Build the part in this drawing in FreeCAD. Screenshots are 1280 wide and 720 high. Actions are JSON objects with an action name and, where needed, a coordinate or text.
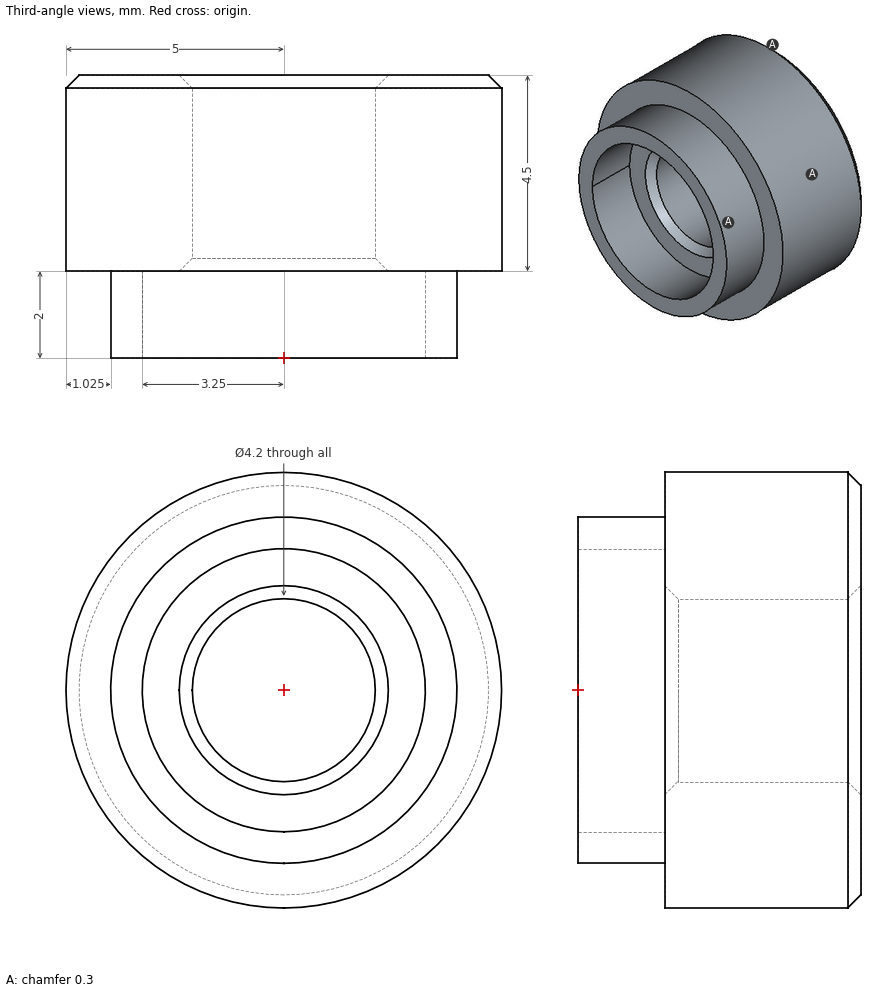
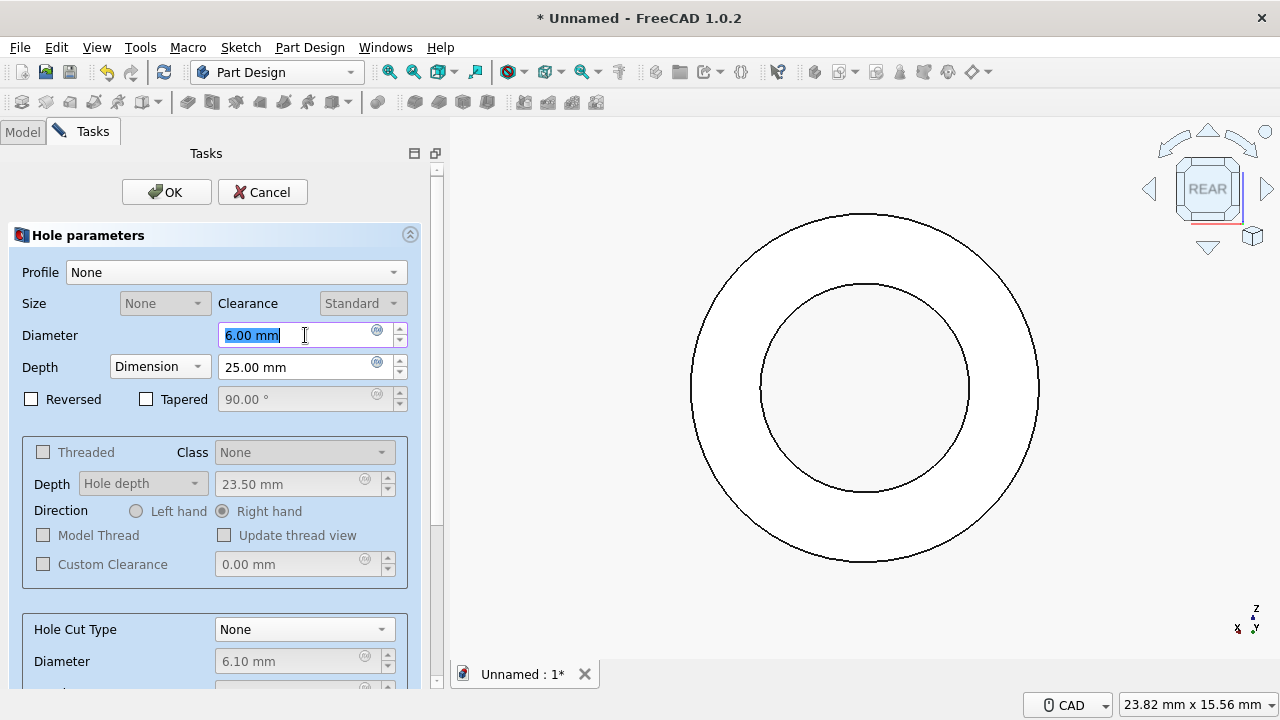
{"action": "type", "text": "4.2"}
{"action": "key", "text": "Tab"}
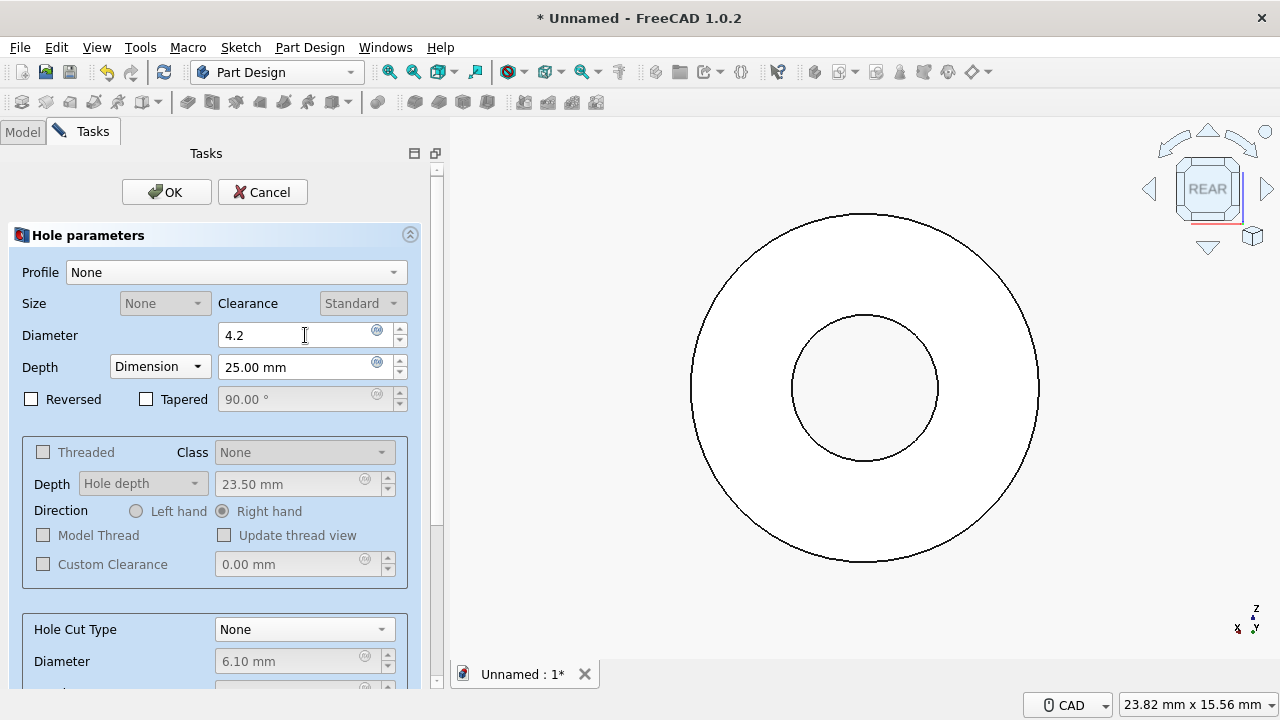
{"action": "left_click", "coordinate": [161, 366]}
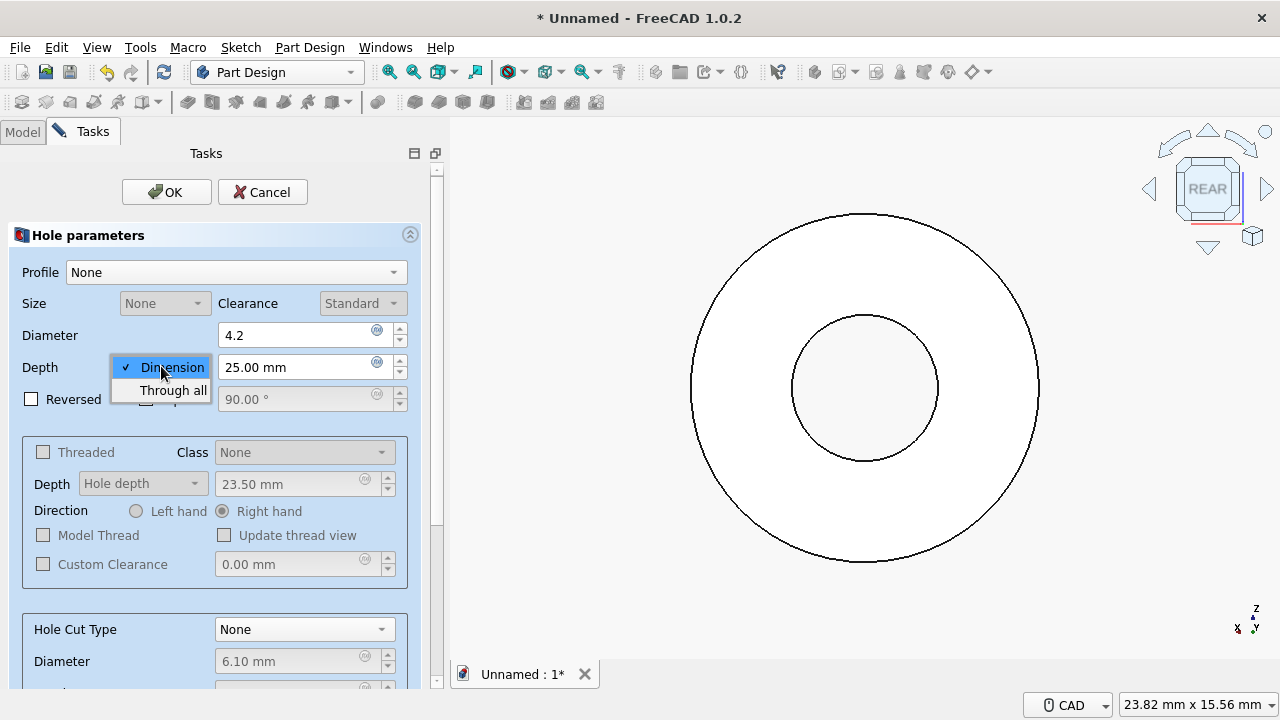
{"action": "left_click", "coordinate": [160, 390]}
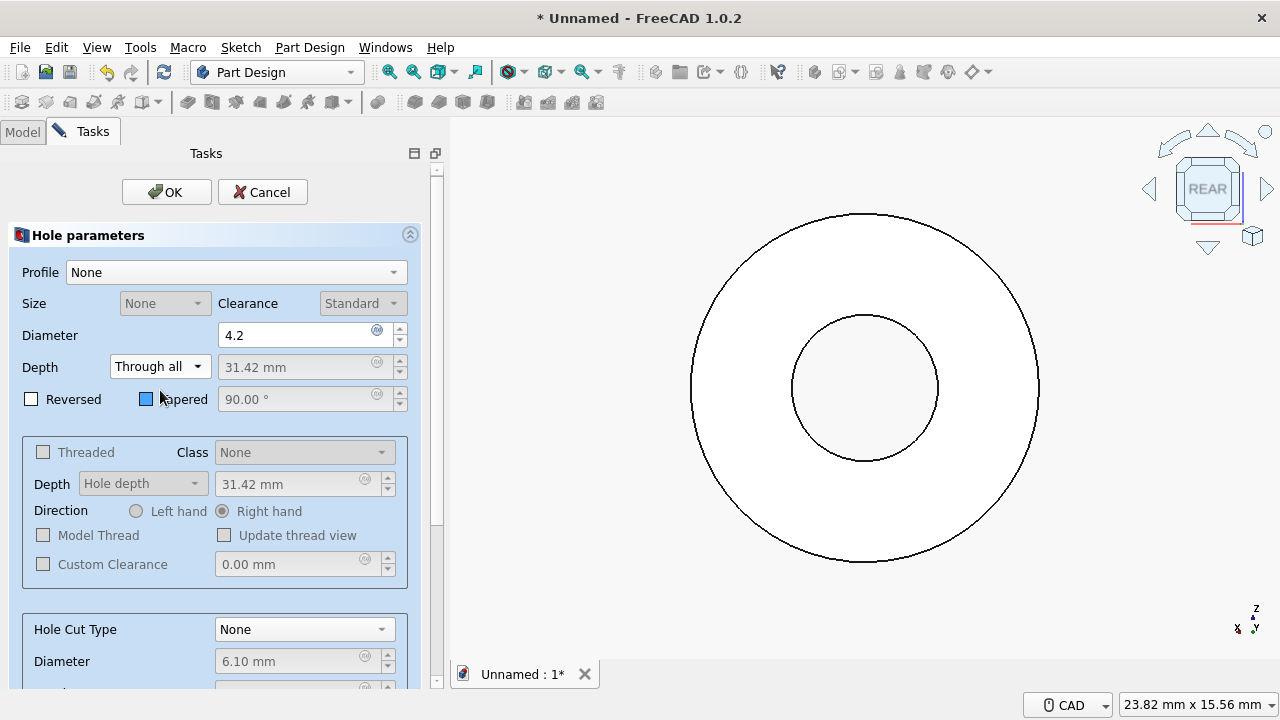
{"action": "left_click", "coordinate": [167, 192]}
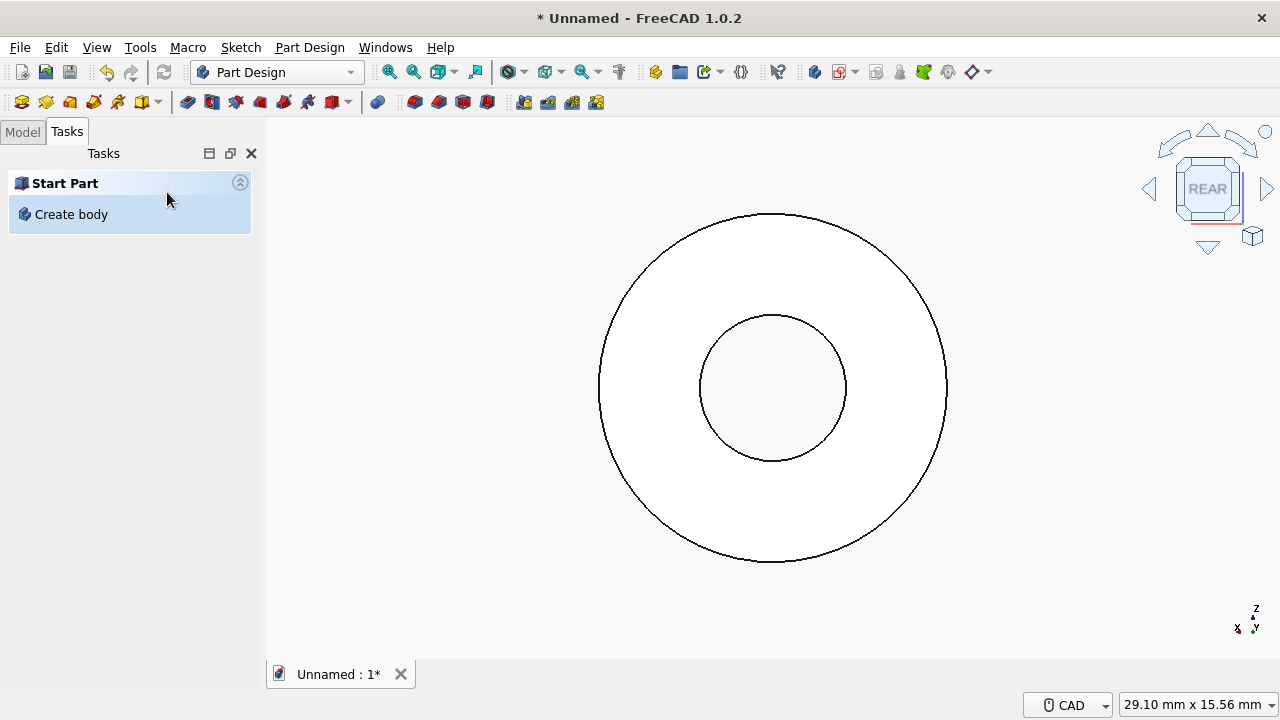
{"action": "left_click", "coordinate": [750, 457]}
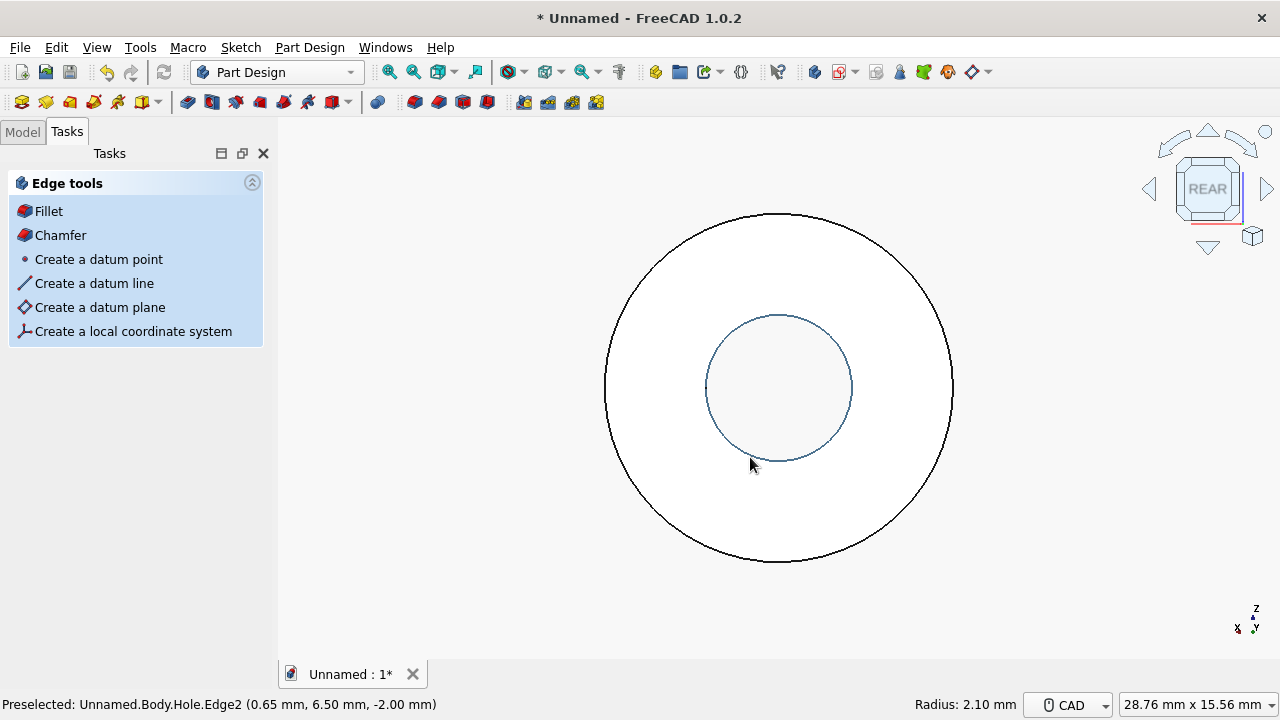
{"action": "left_click", "coordinate": [638, 285], "text": "ctrl"}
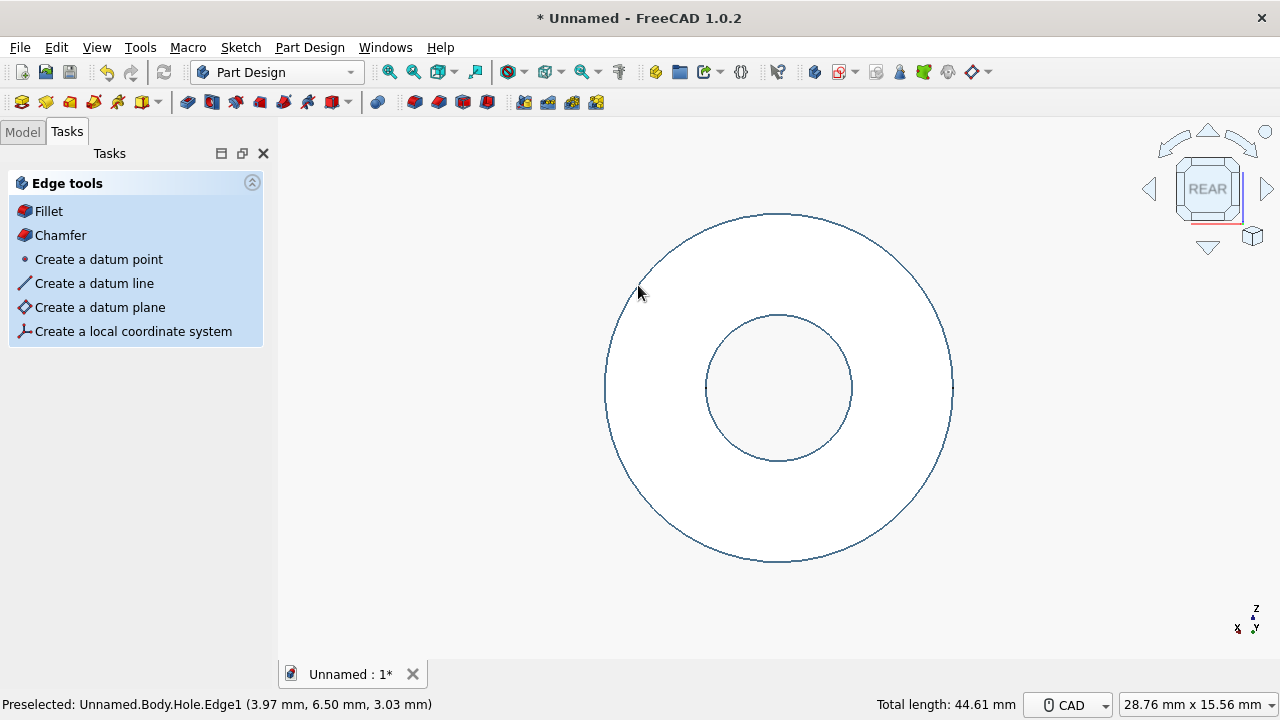
{"action": "key", "text": "0"}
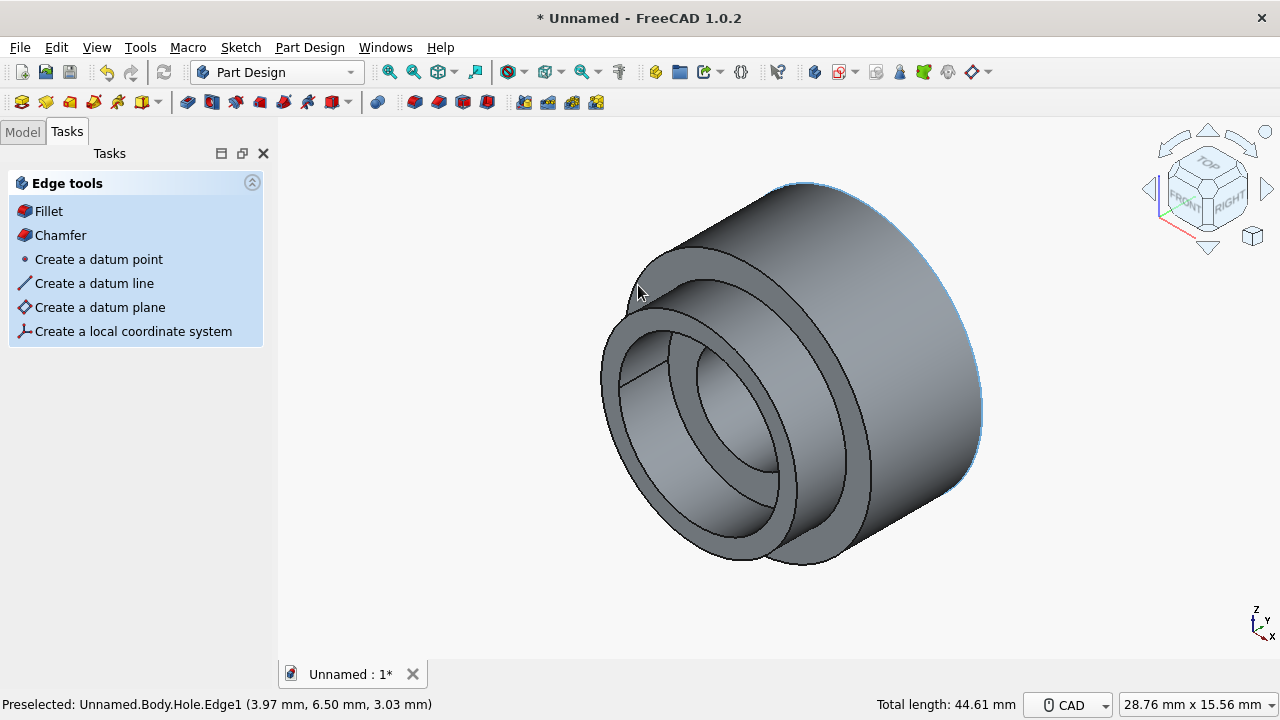
{"action": "left_click", "coordinate": [697, 375], "text": "ctrl"}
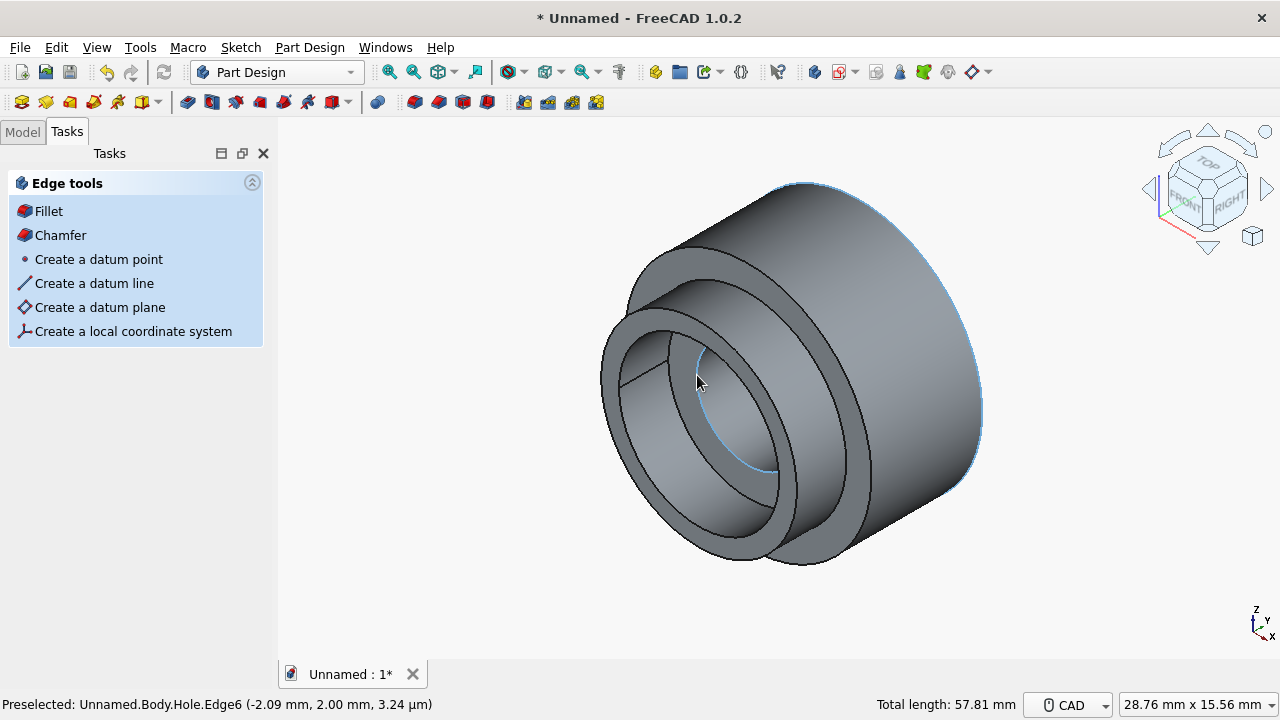
{"action": "left_click", "coordinate": [440, 102]}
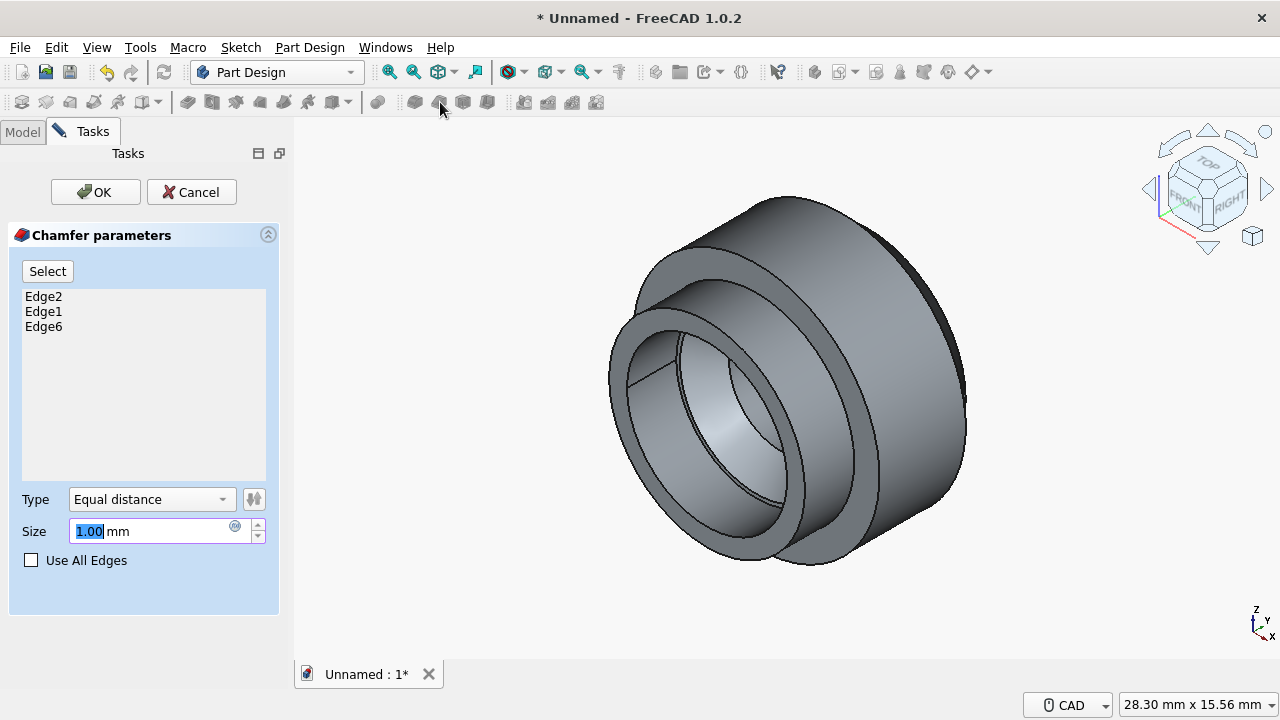
{"action": "type", "text": "0.3"}
{"action": "key", "text": "Tab"}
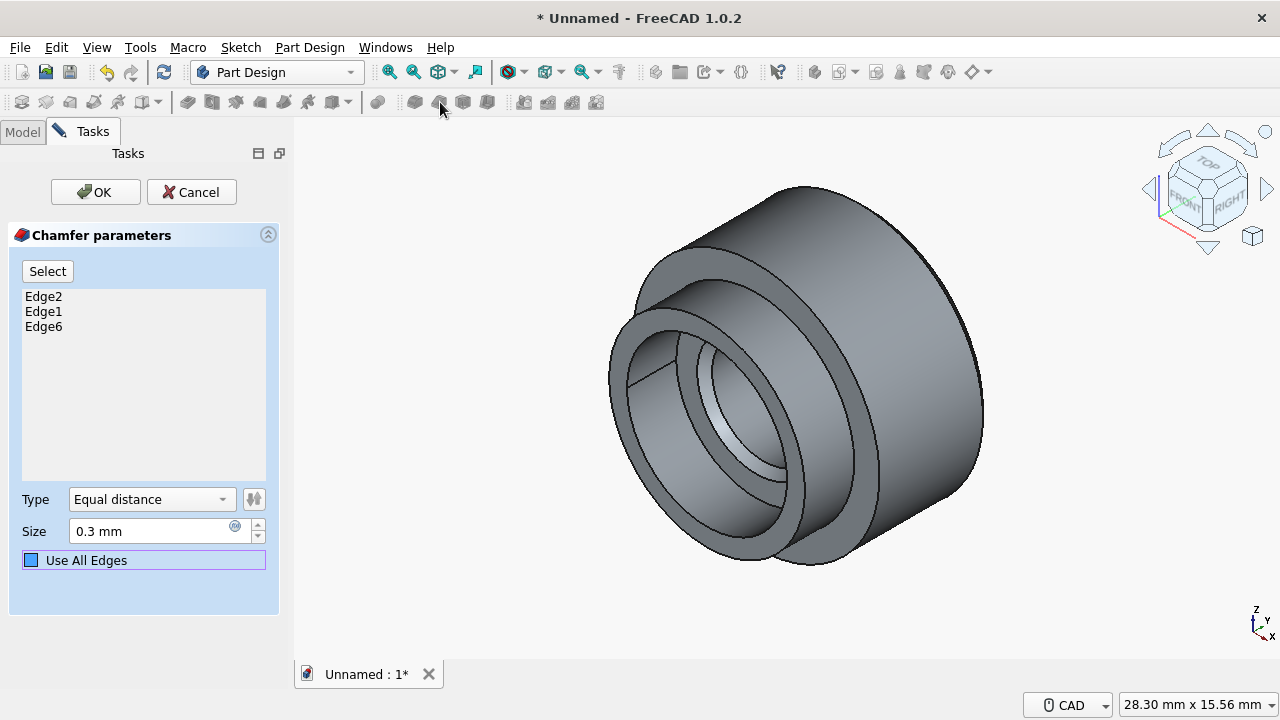
{"action": "left_click", "coordinate": [96, 192]}